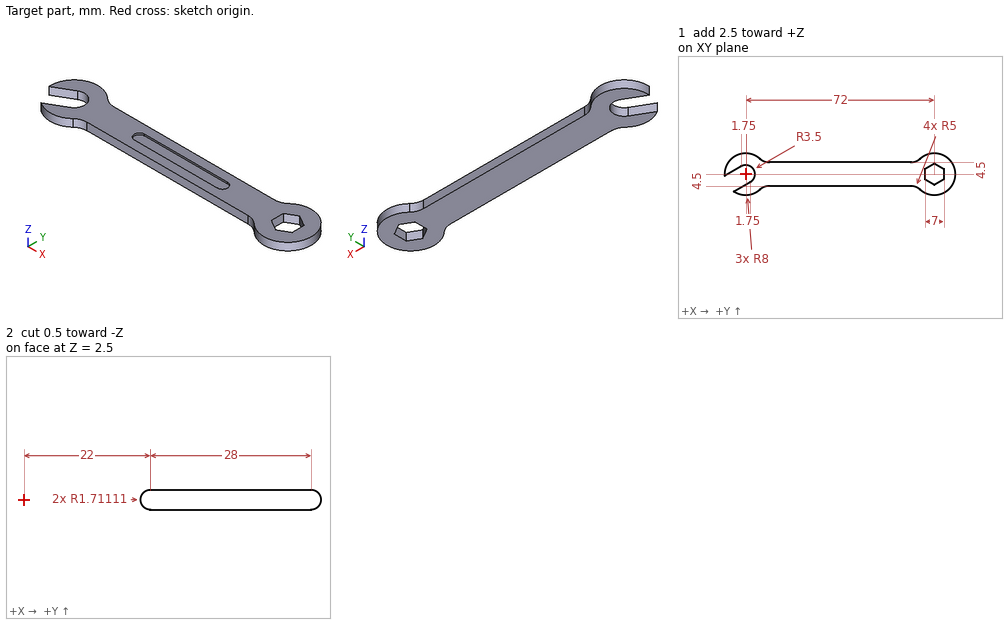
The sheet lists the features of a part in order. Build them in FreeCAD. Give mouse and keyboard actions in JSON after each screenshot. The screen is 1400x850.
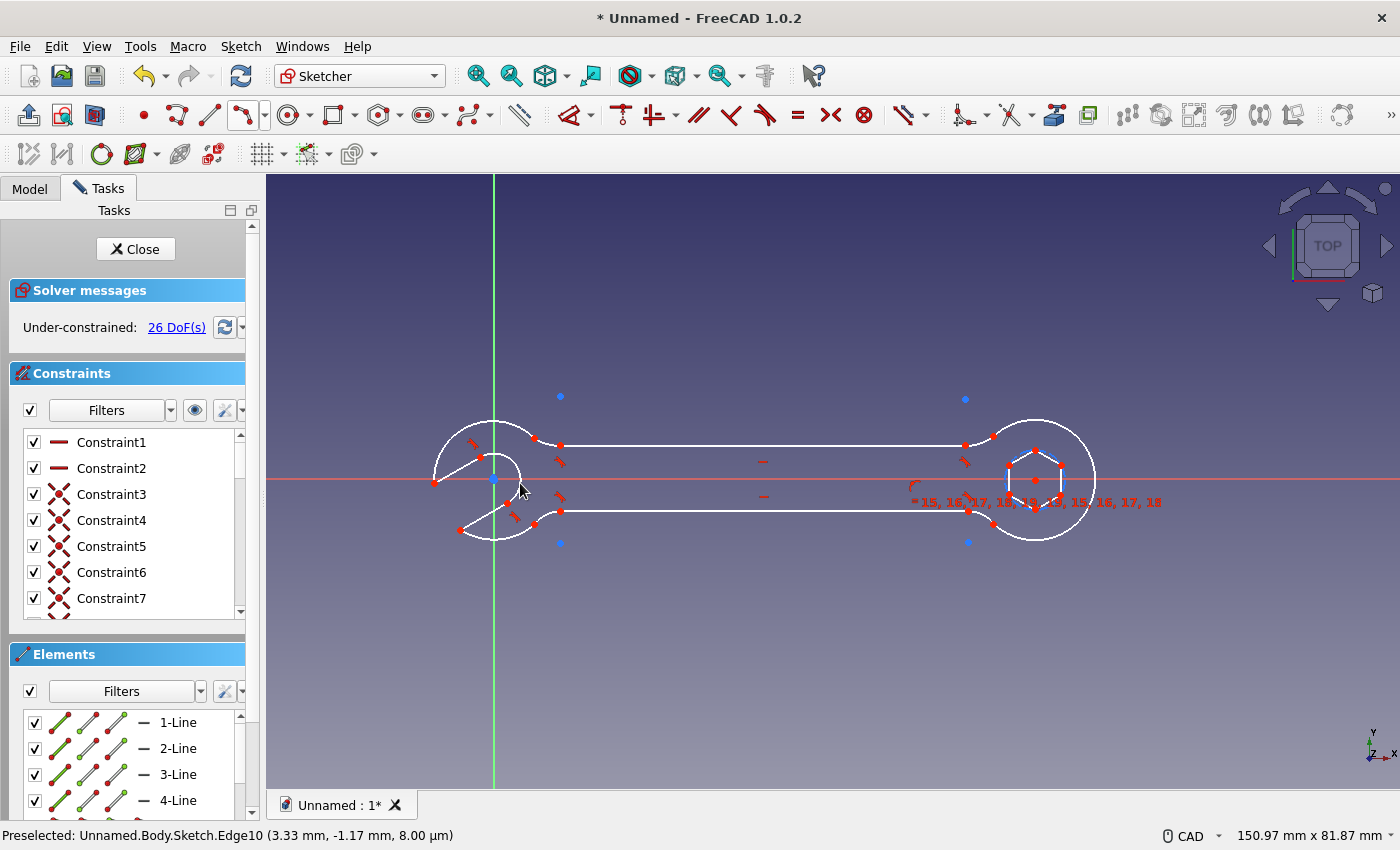
{"action": "left_click", "coordinate": [983, 515]}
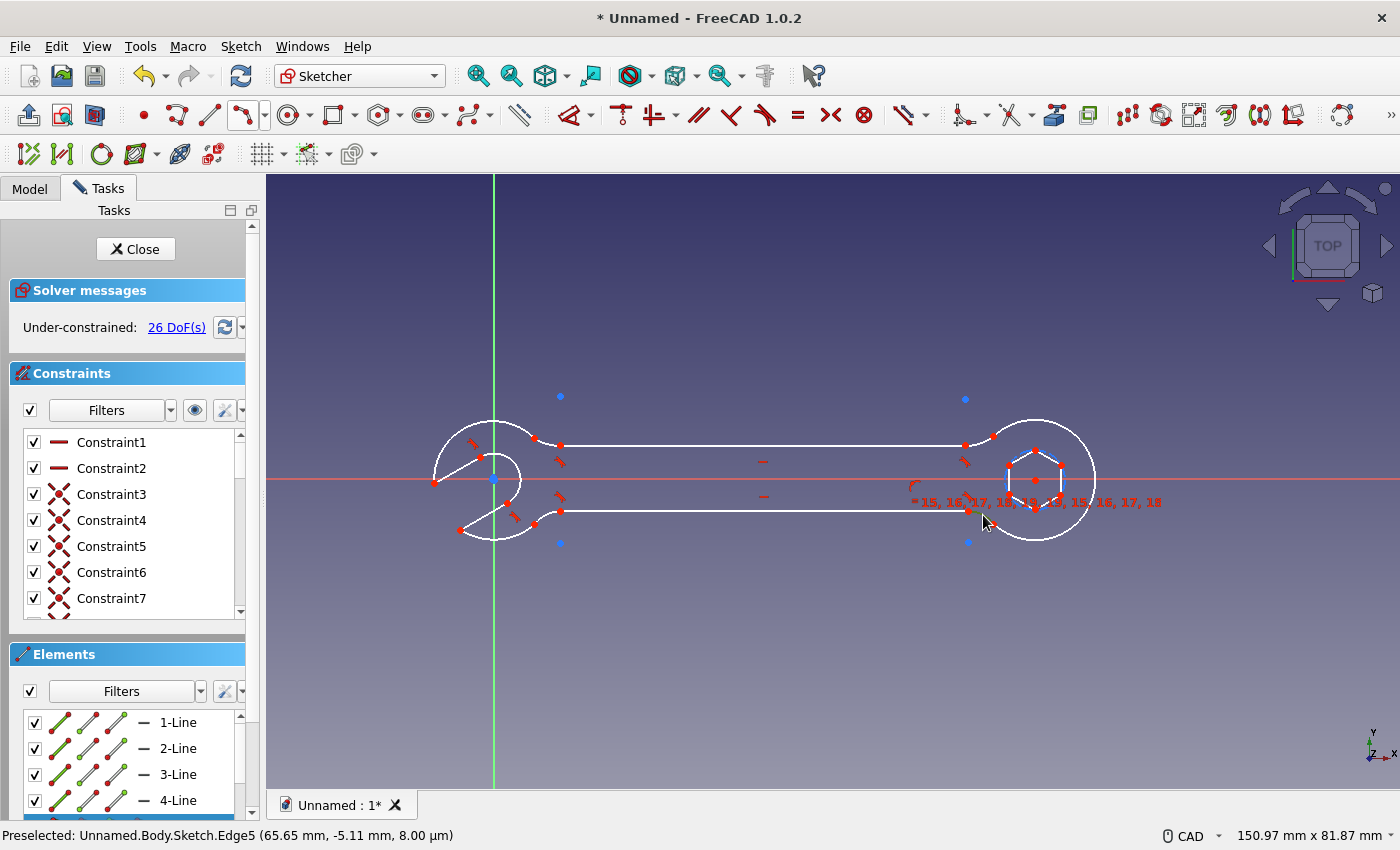
{"action": "left_click", "coordinate": [1071, 528]}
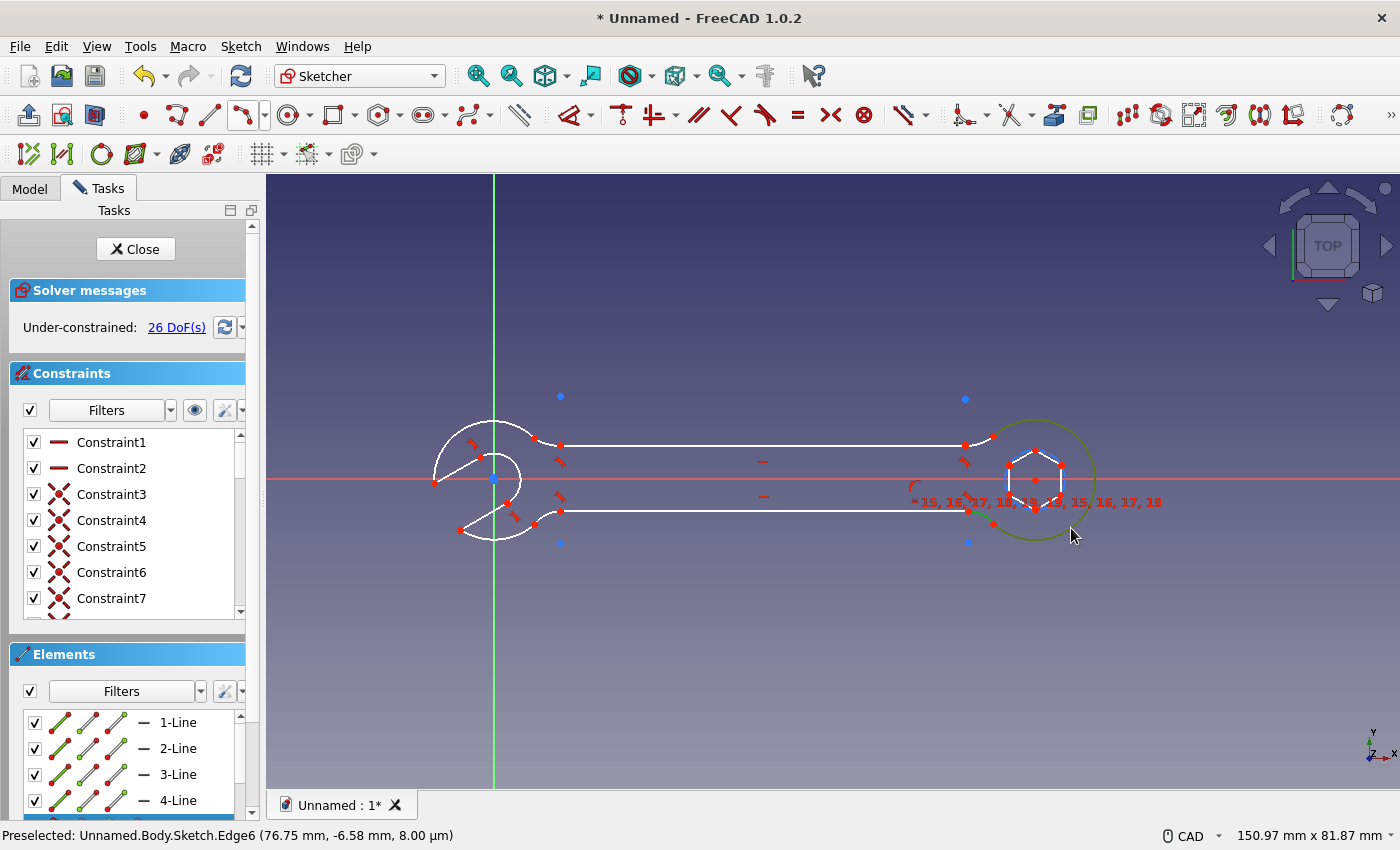
{"action": "left_click", "coordinate": [765, 116]}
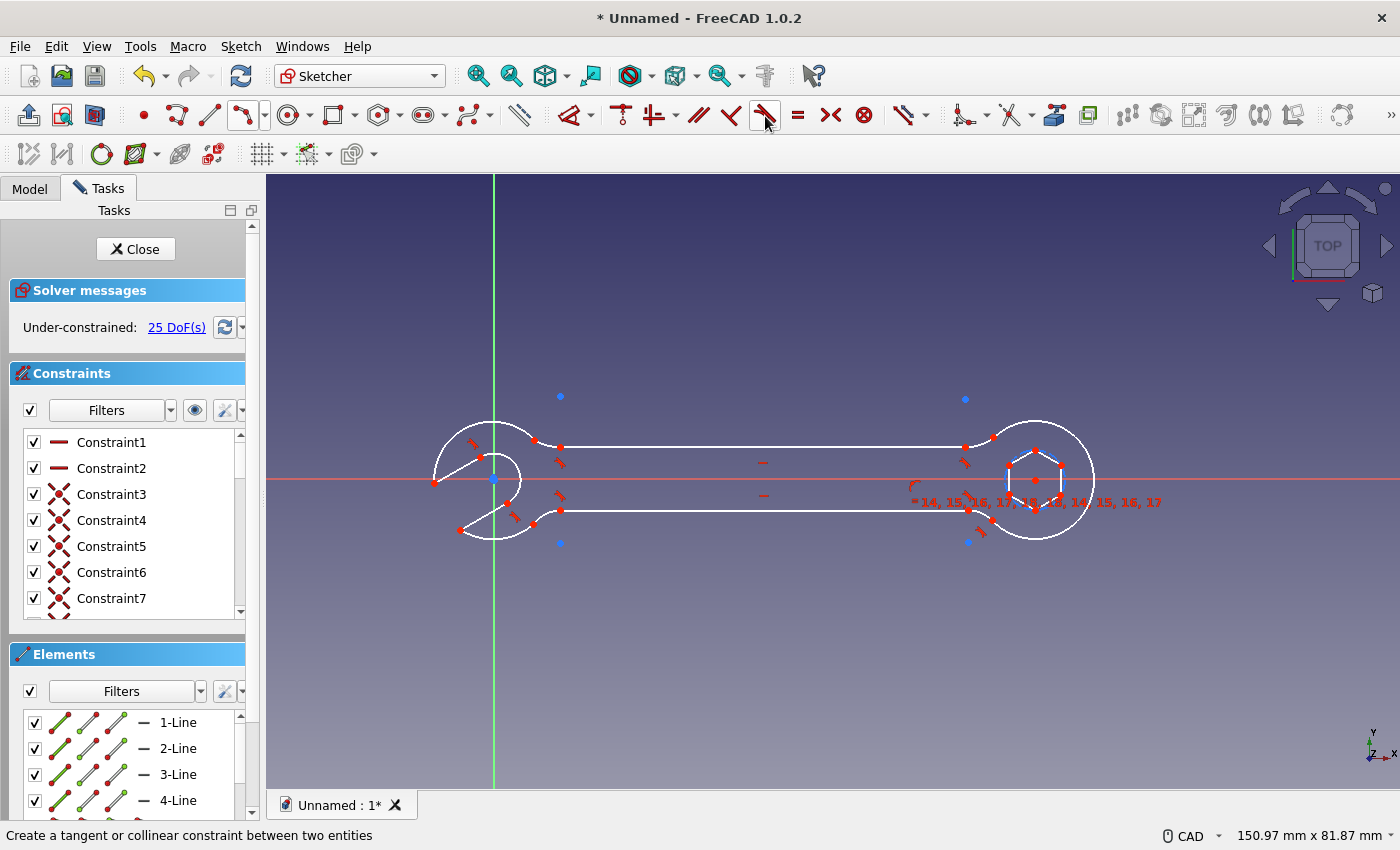
{"action": "left_click", "coordinate": [1069, 529]}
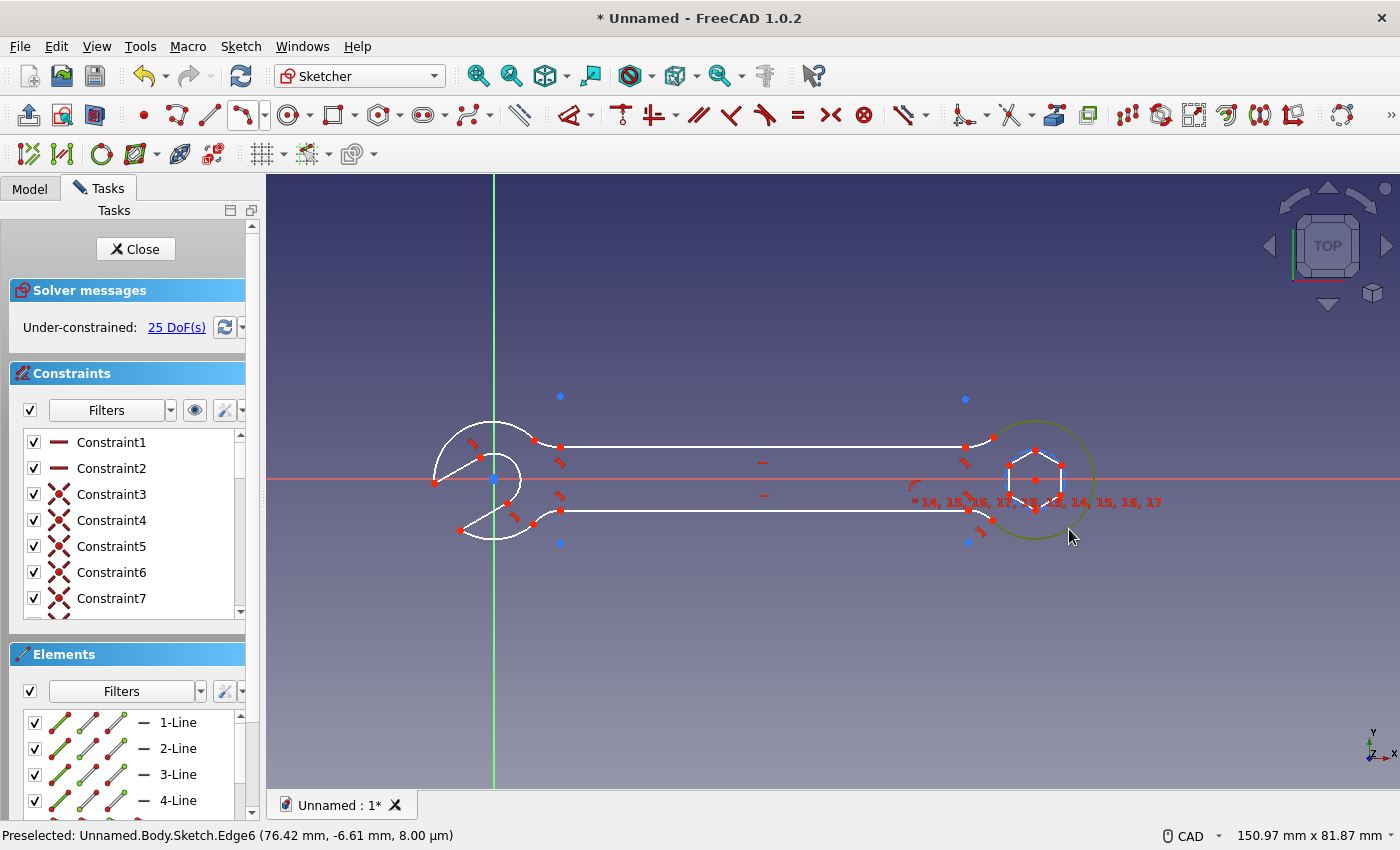
{"action": "scroll", "coordinate": [974, 446], "scroll_direction": "up", "scroll_amount": 3}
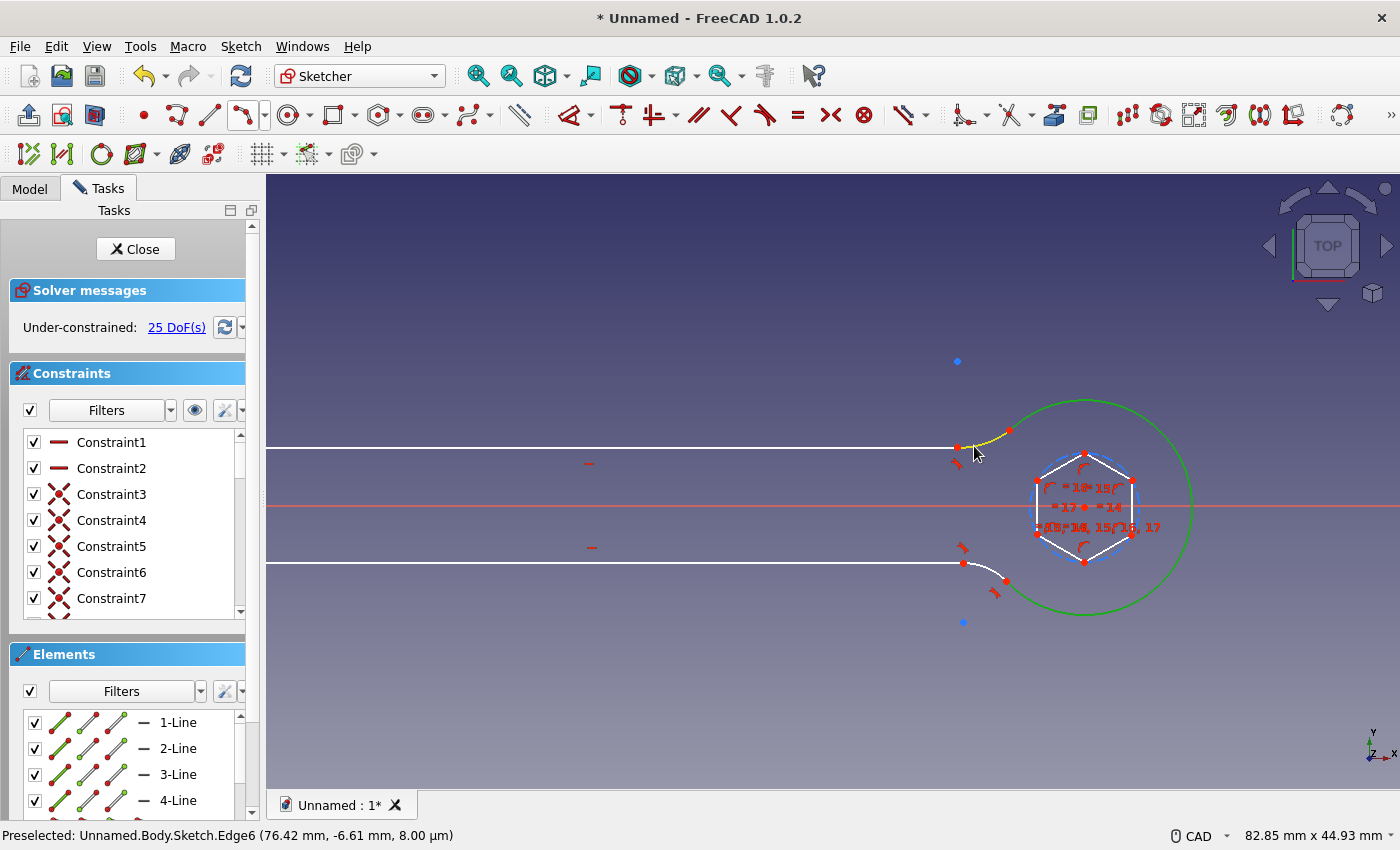
{"action": "left_click", "coordinate": [974, 446]}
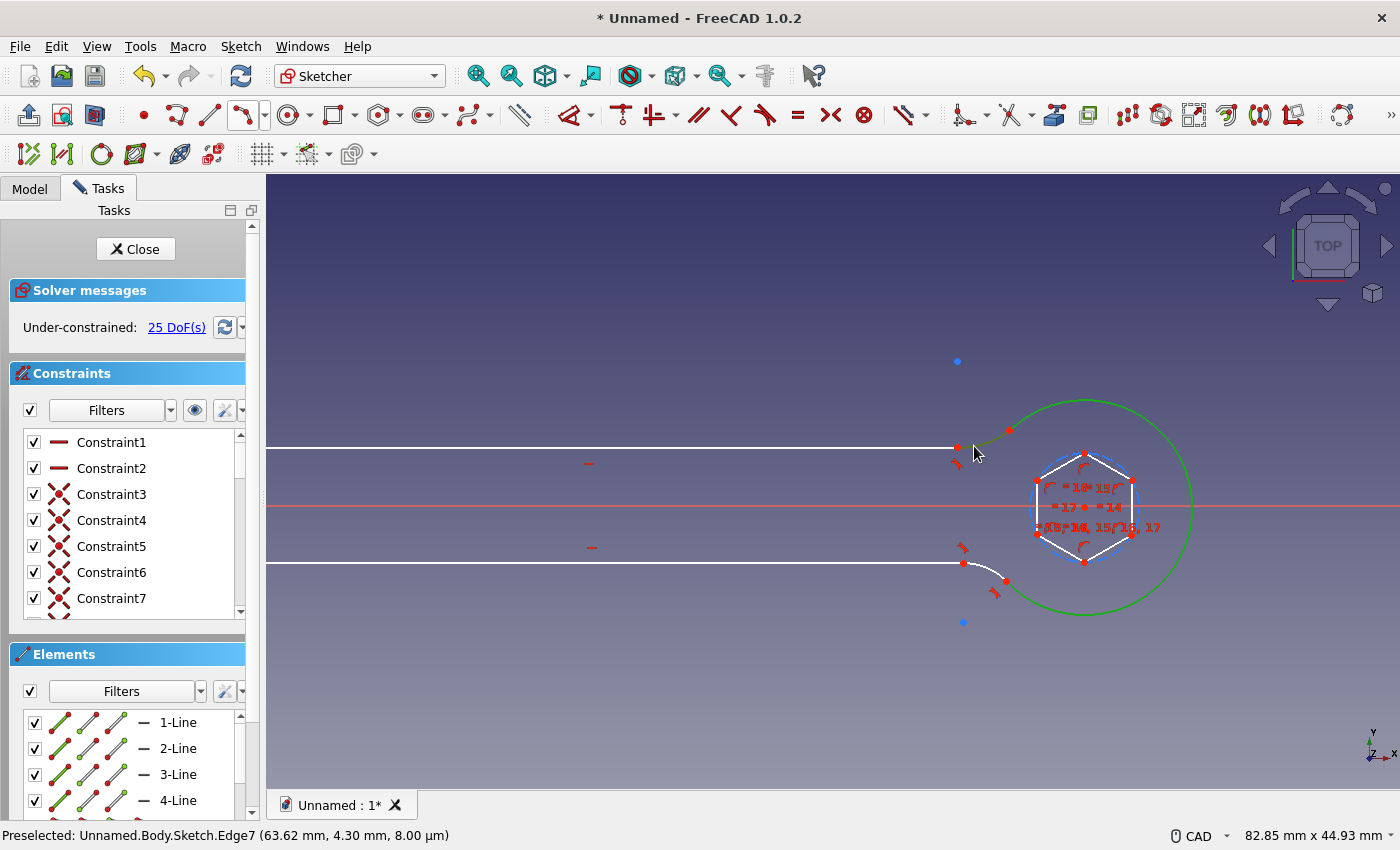
{"action": "key", "text": "t"}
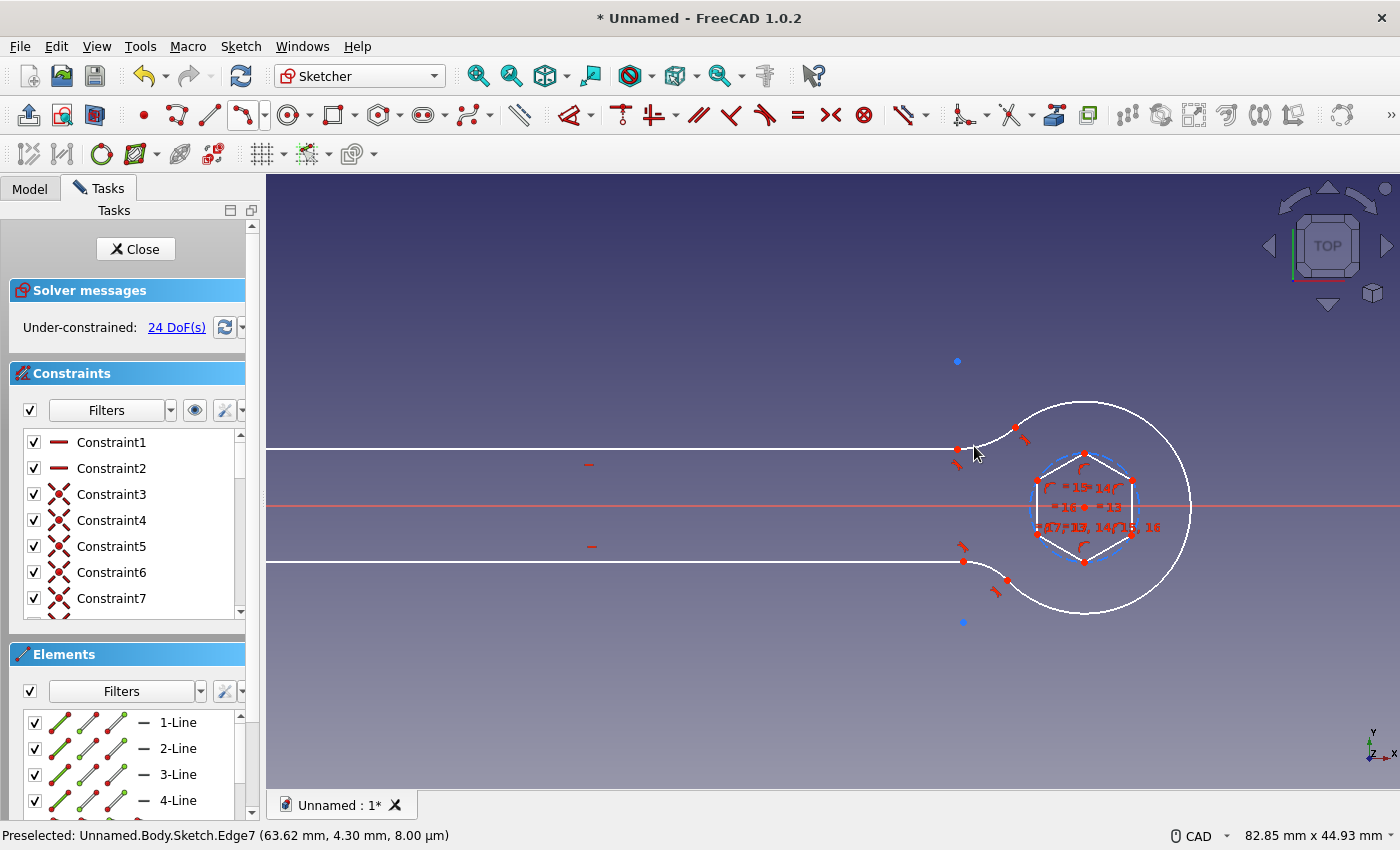
{"action": "scroll", "coordinate": [974, 446], "scroll_direction": "down", "scroll_amount": 3}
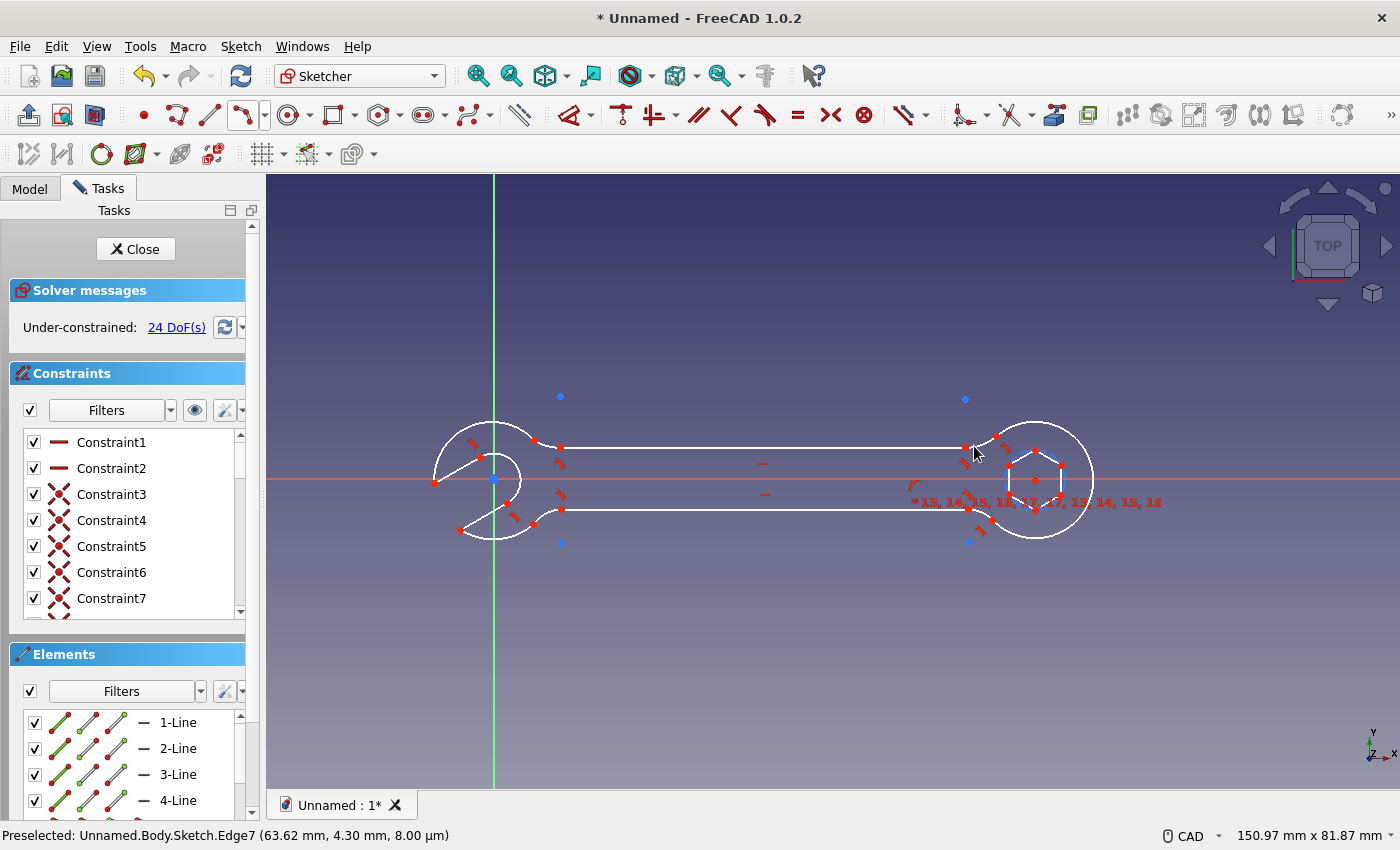
{"action": "scroll", "coordinate": [542, 444], "scroll_direction": "up", "scroll_amount": 3}